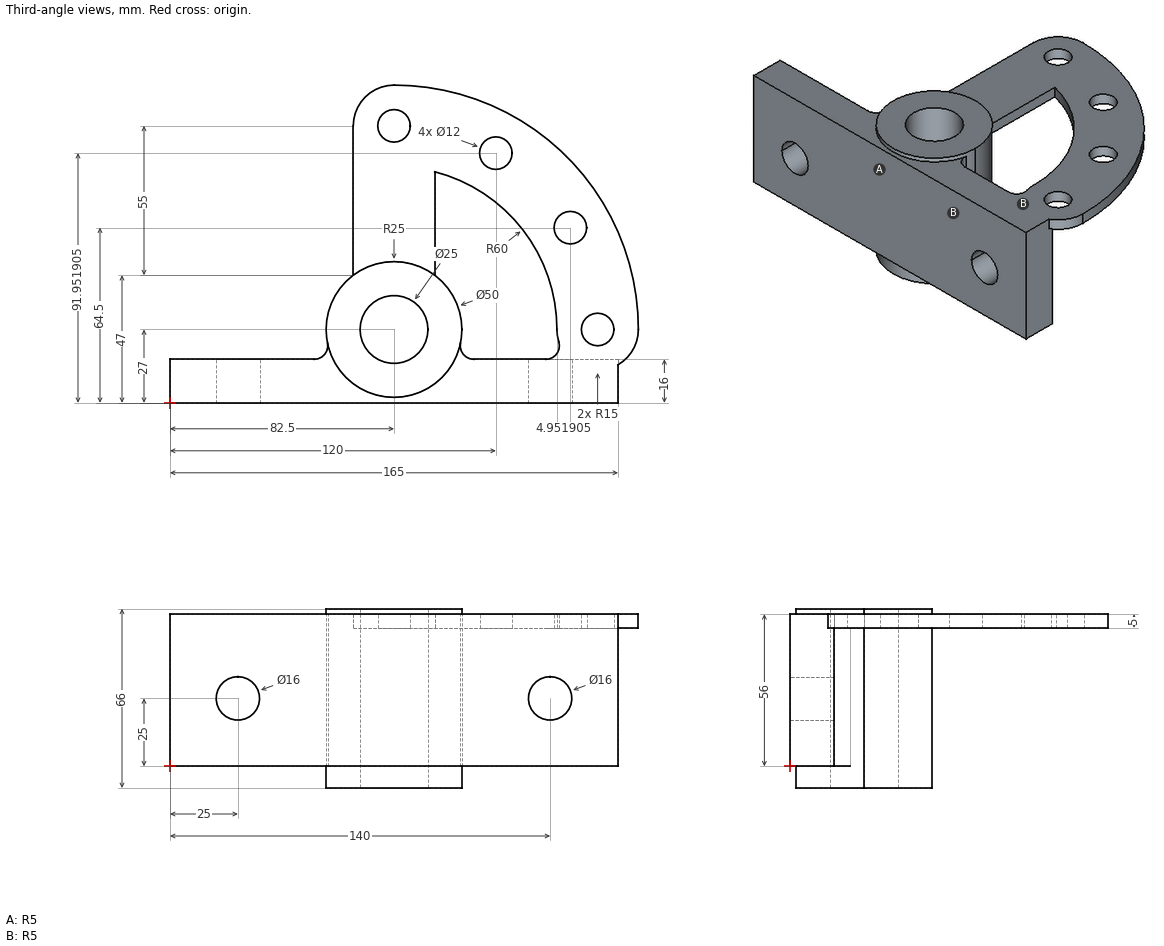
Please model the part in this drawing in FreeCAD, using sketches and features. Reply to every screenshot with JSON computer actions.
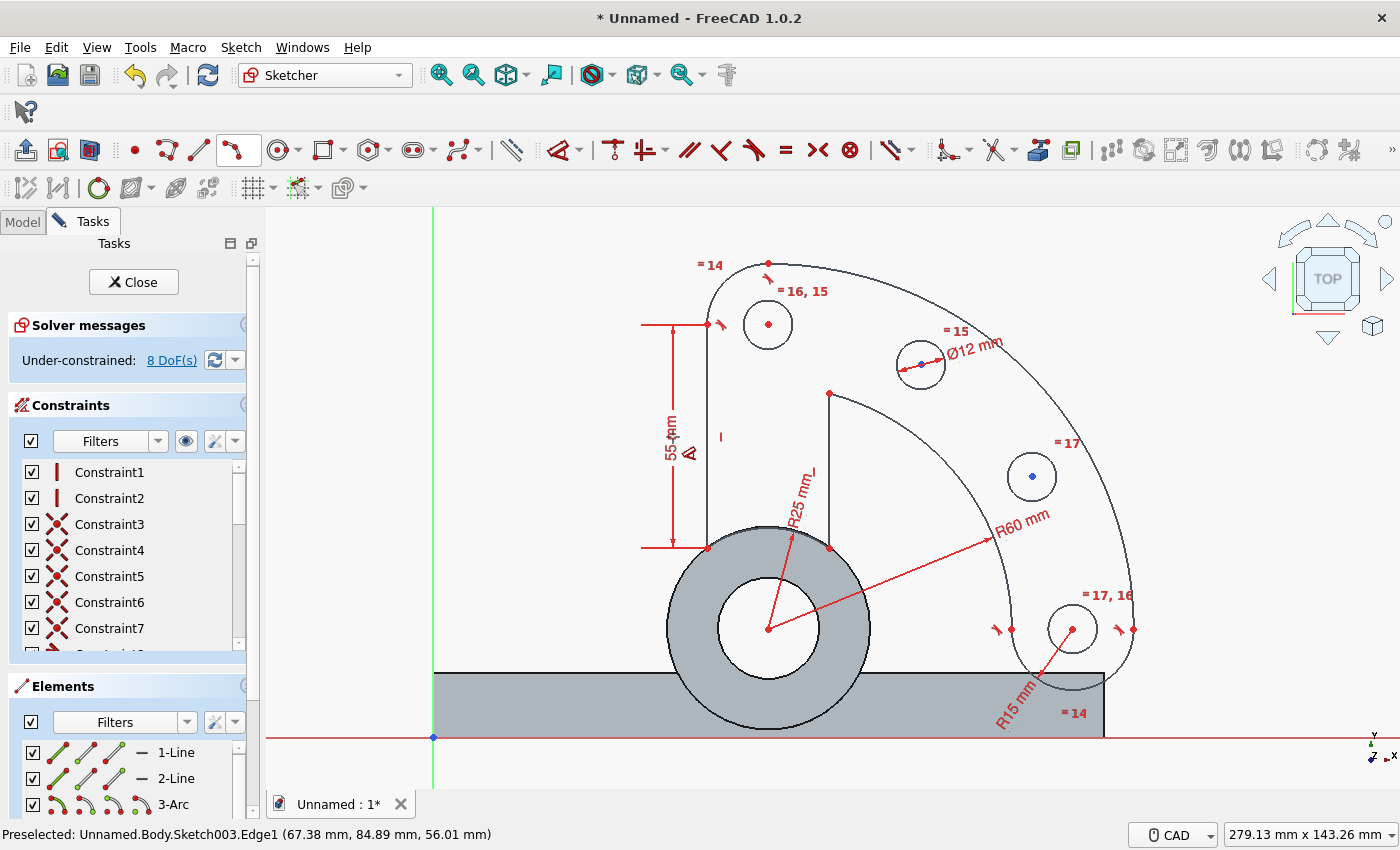
{"action": "left_click", "coordinate": [1073, 629]}
{"action": "left_click", "coordinate": [399, 684]}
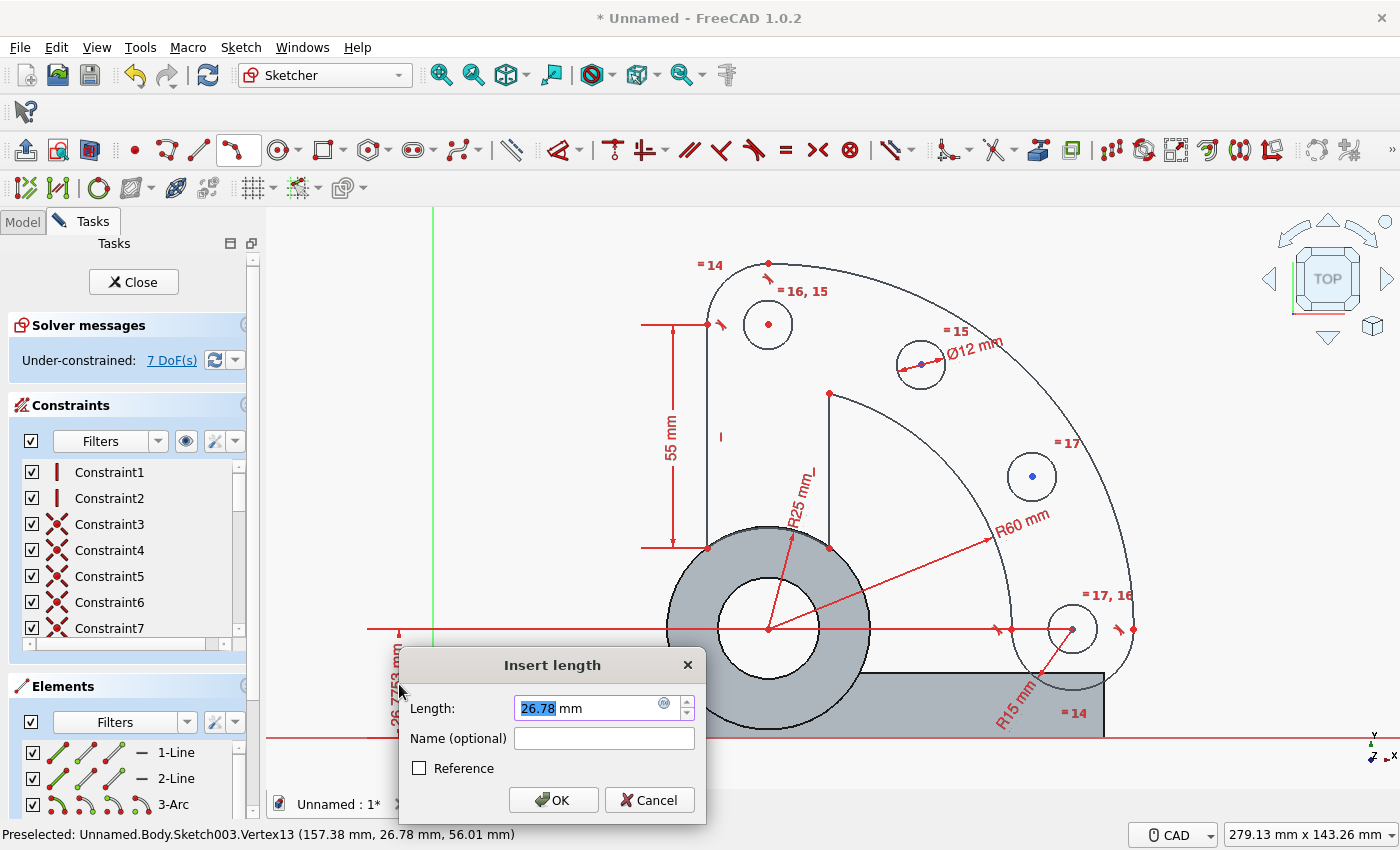
{"action": "type", "text": "27"}
{"action": "key", "text": "Return"}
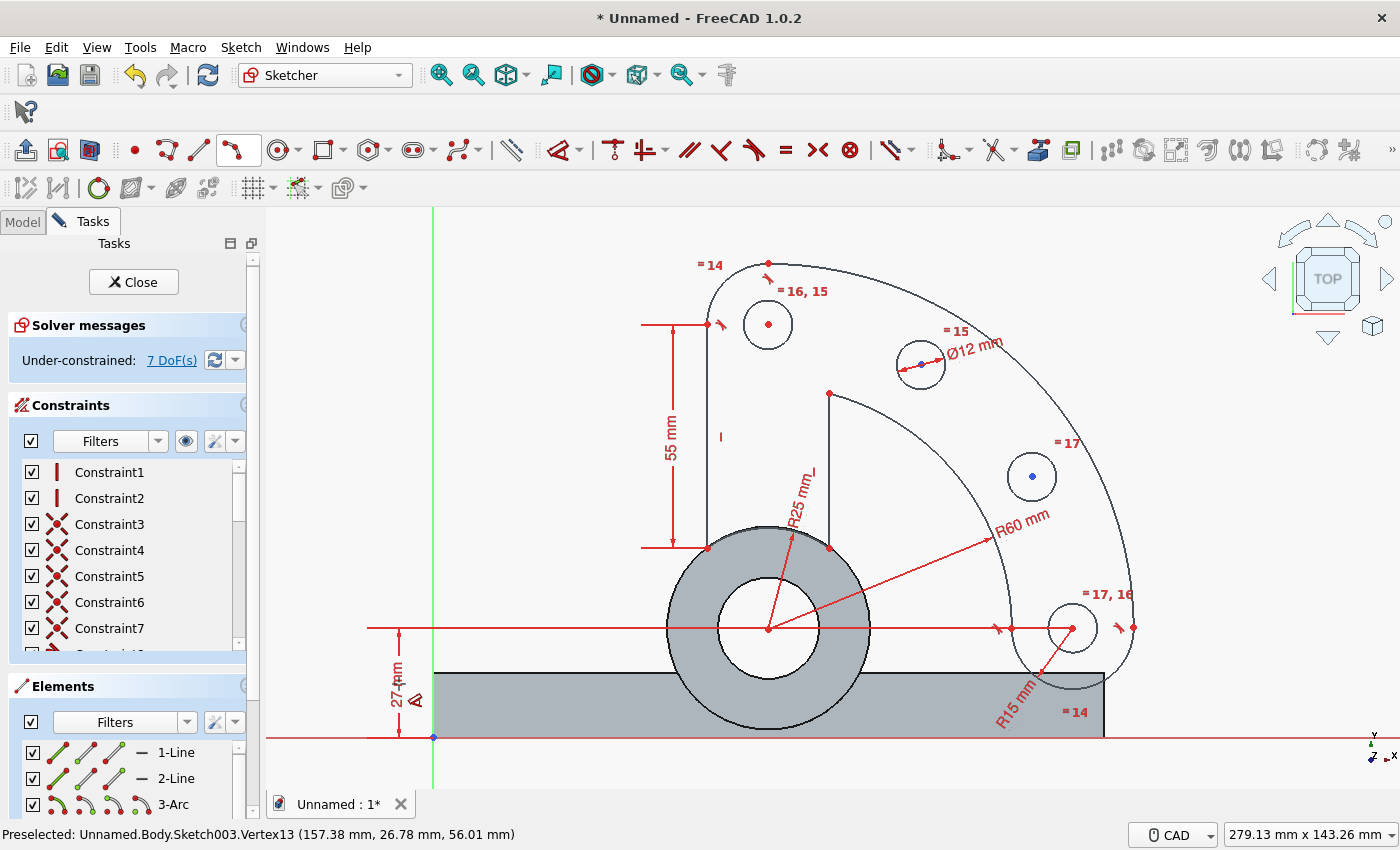
{"action": "left_click", "coordinate": [707, 548]}
{"action": "left_click", "coordinate": [399, 643]}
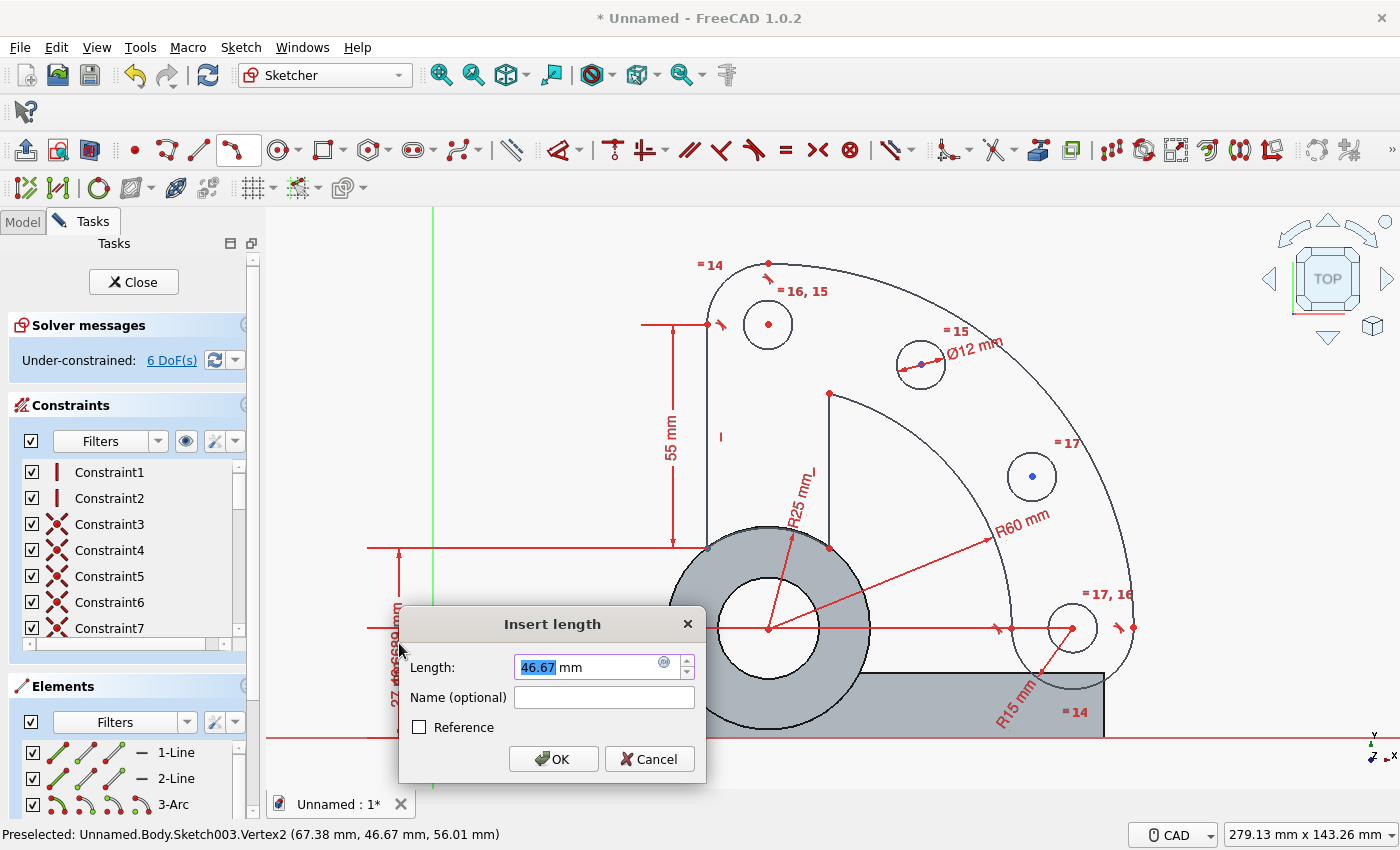
{"action": "type", "text": "47"}
{"action": "key", "text": "Return"}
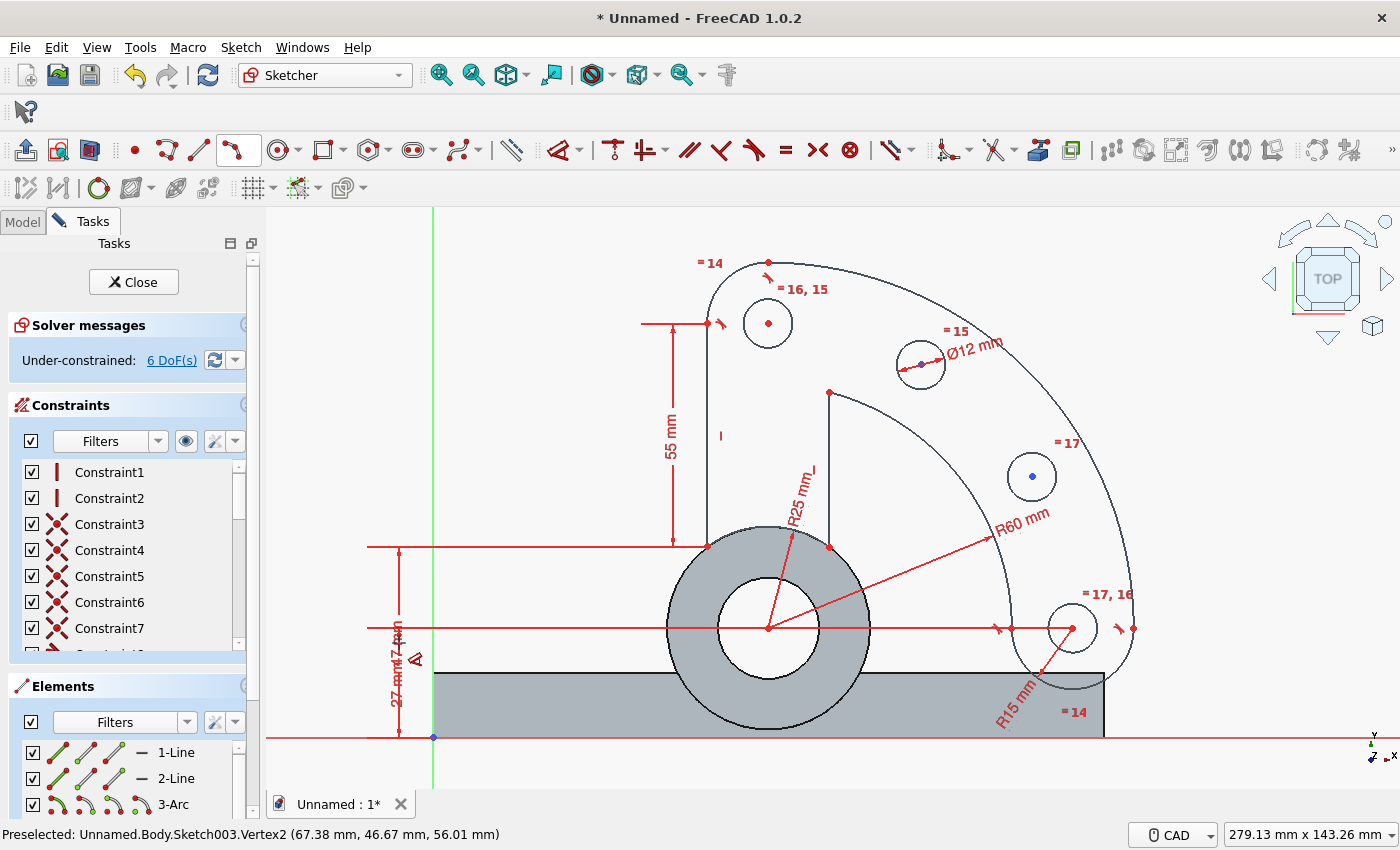
{"action": "left_click", "coordinate": [829, 547]}
{"action": "left_click", "coordinate": [399, 599]}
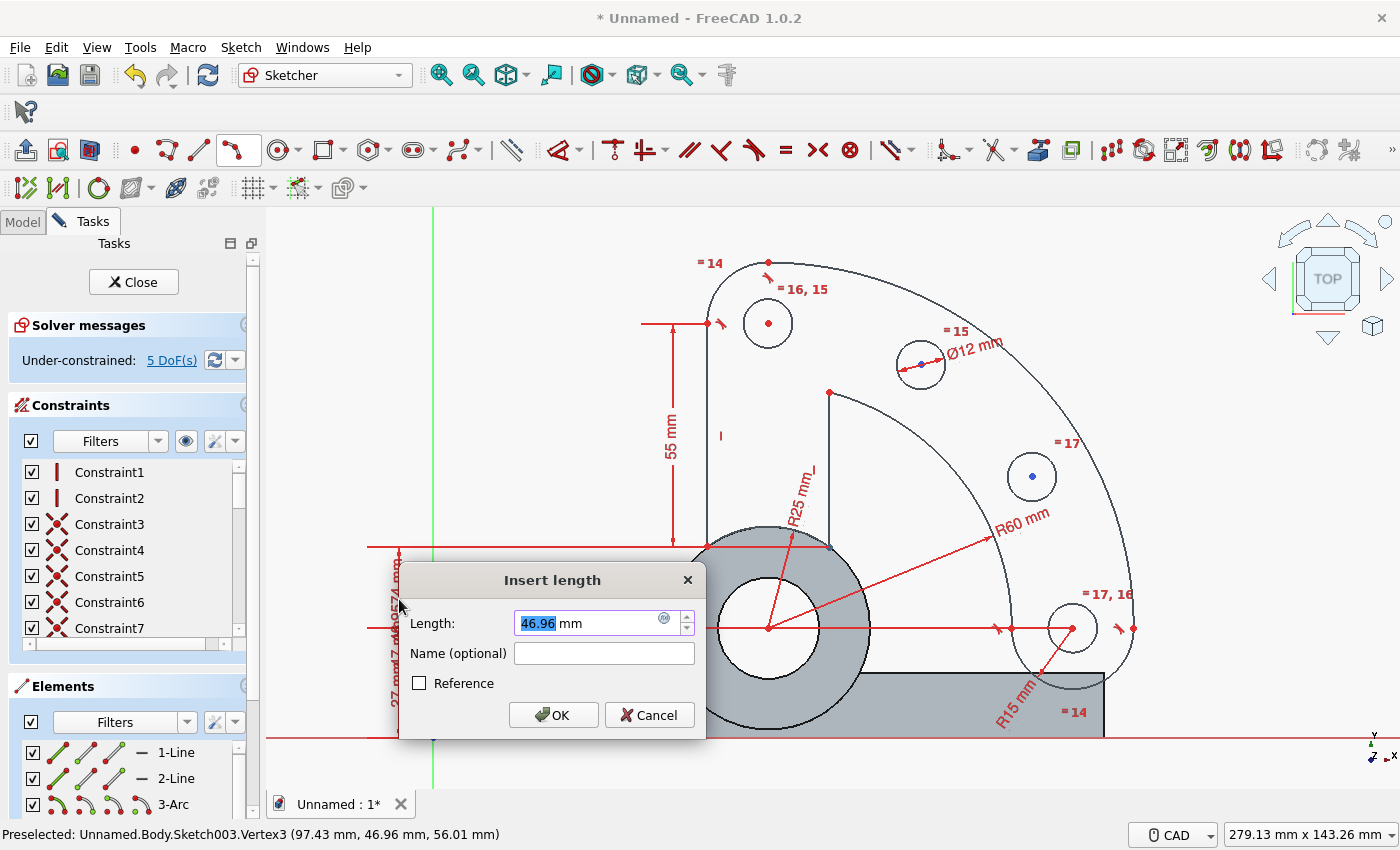
{"action": "type", "text": "47"}
{"action": "key", "text": "Return"}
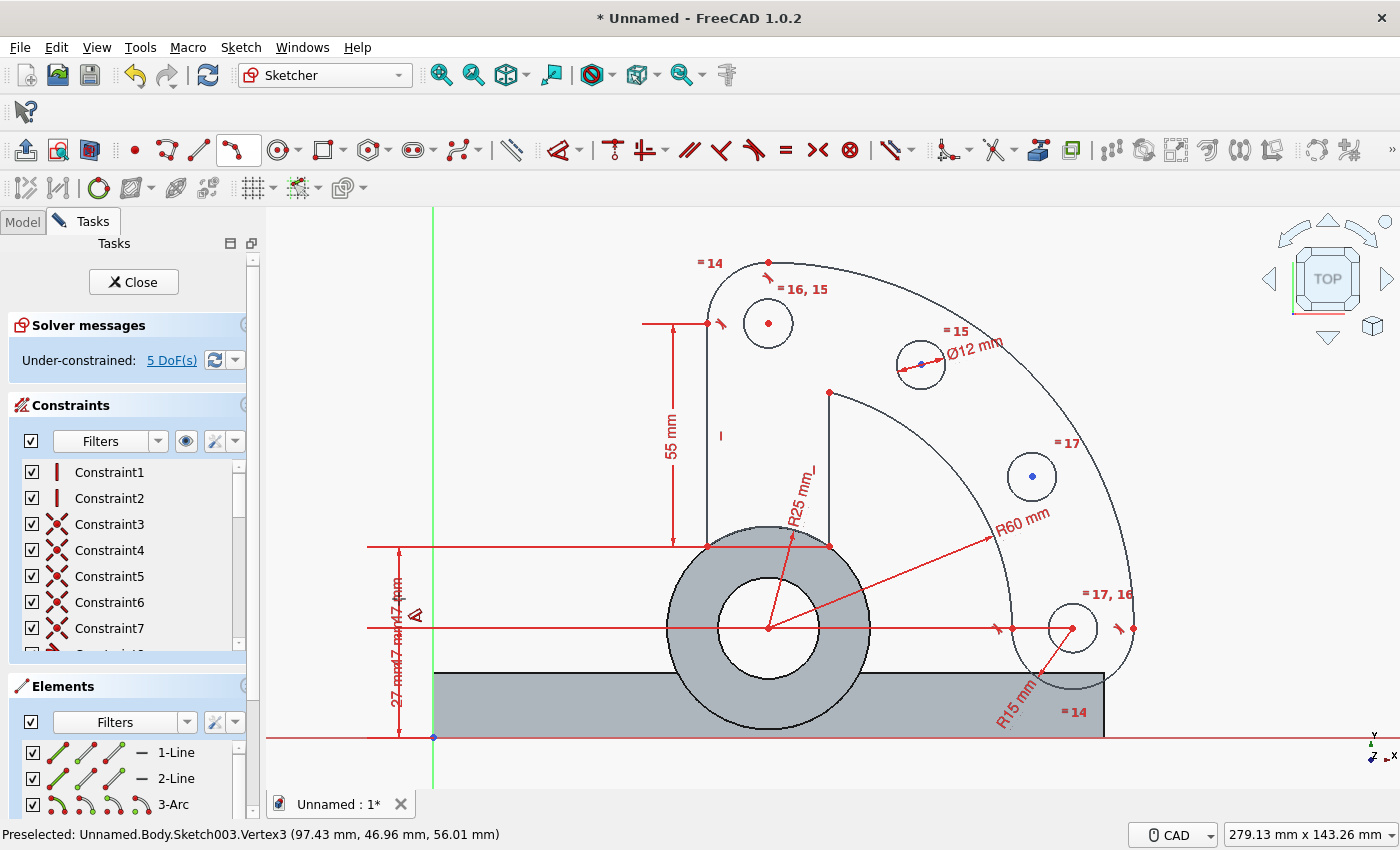
{"action": "left_click", "coordinate": [921, 365]}
{"action": "left_click", "coordinate": [677, 331]}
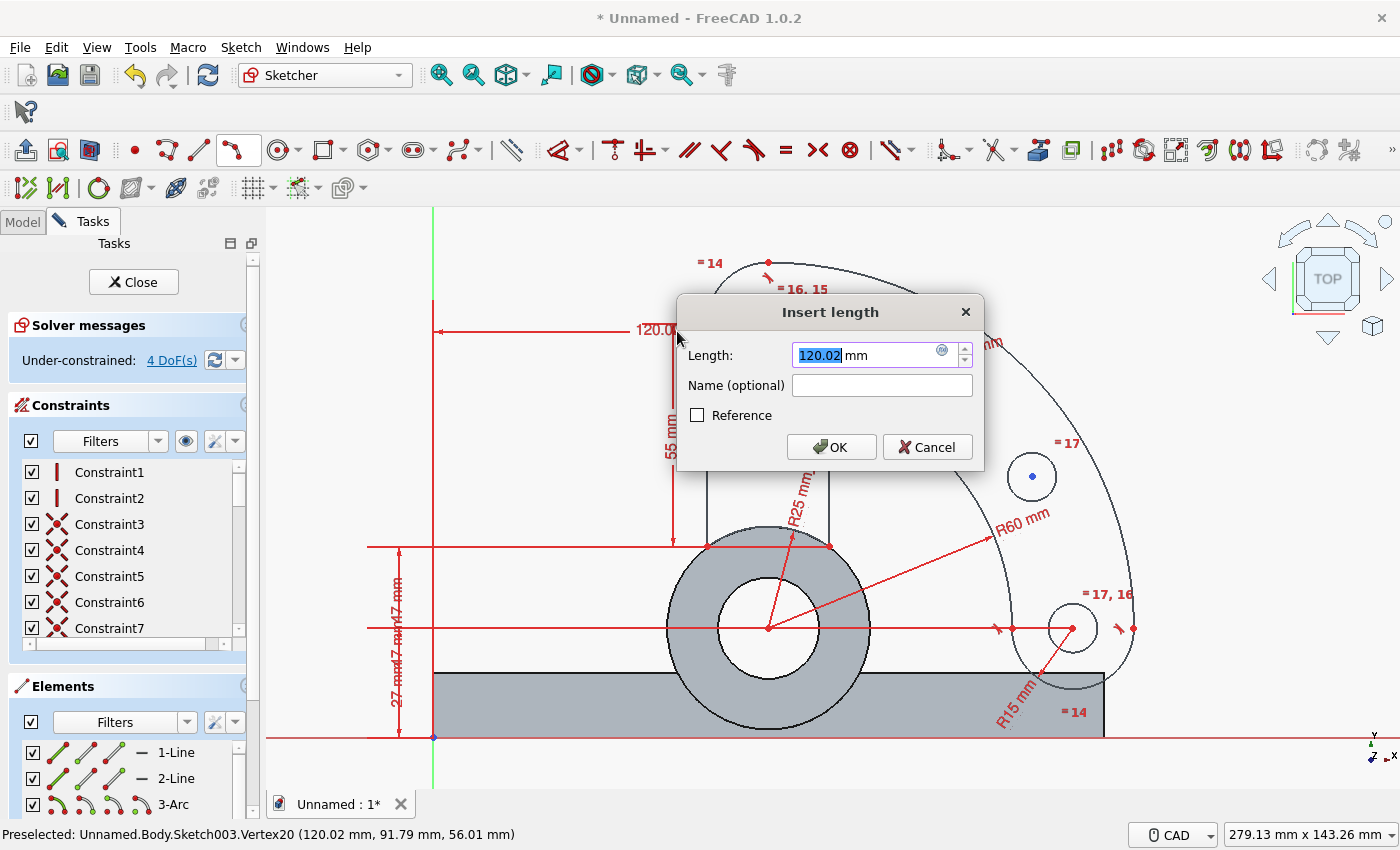
{"action": "type", "text": "120"}
{"action": "key", "text": "Return"}